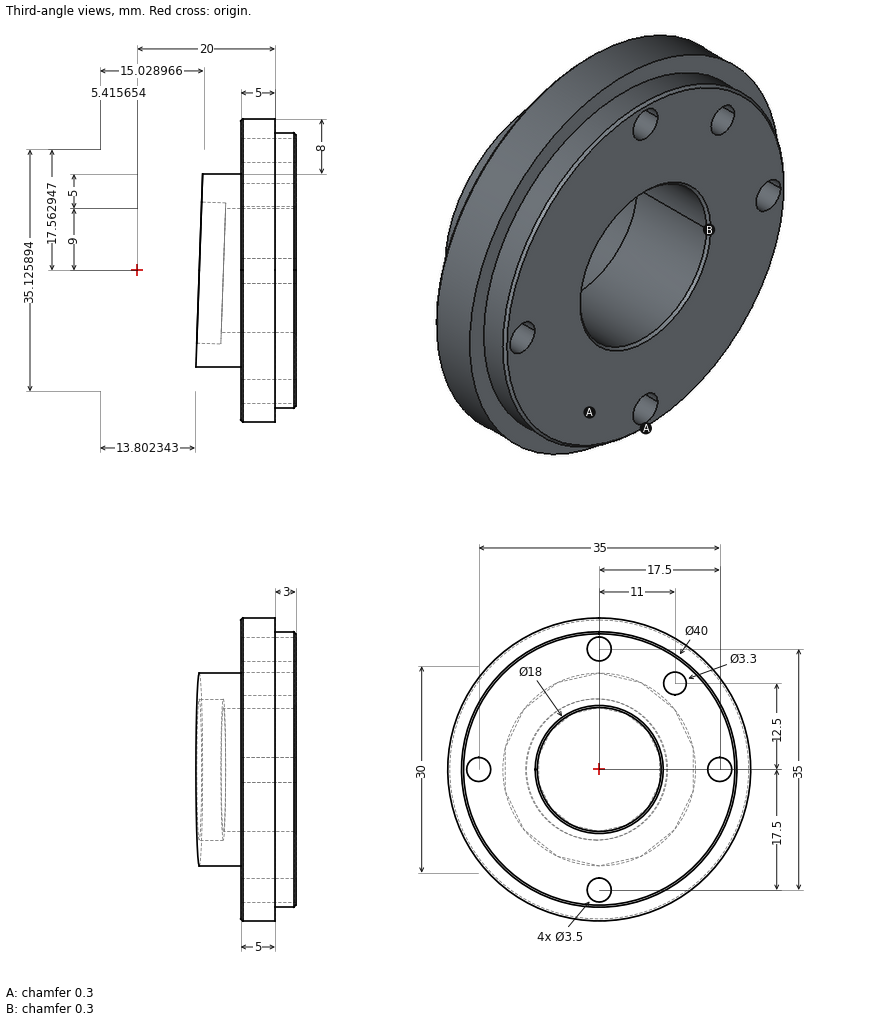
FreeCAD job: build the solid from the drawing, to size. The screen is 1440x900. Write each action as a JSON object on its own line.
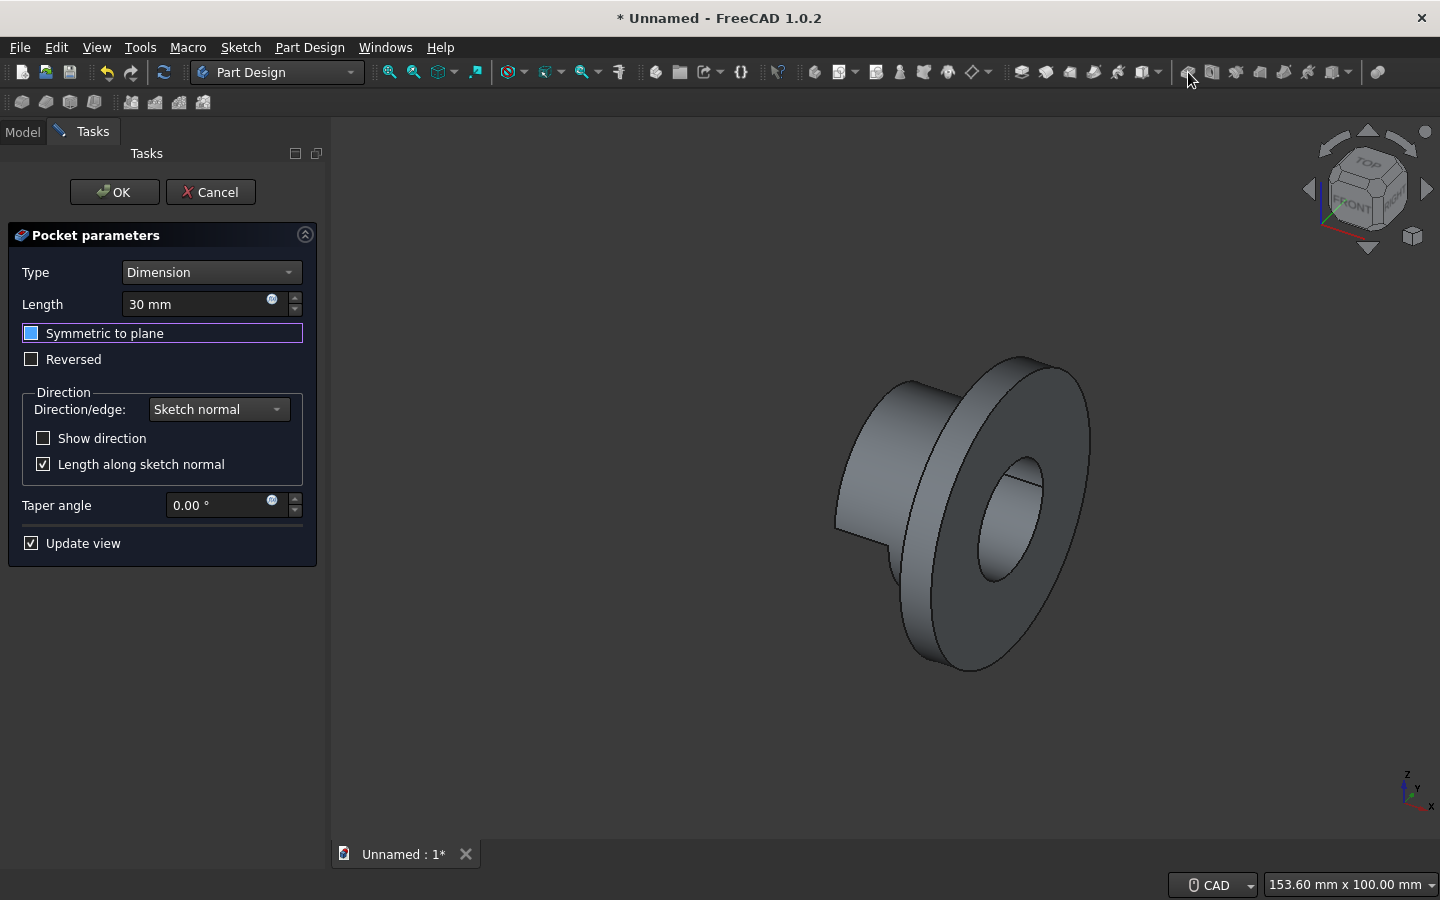
{"action": "left_click", "coordinate": [30, 333]}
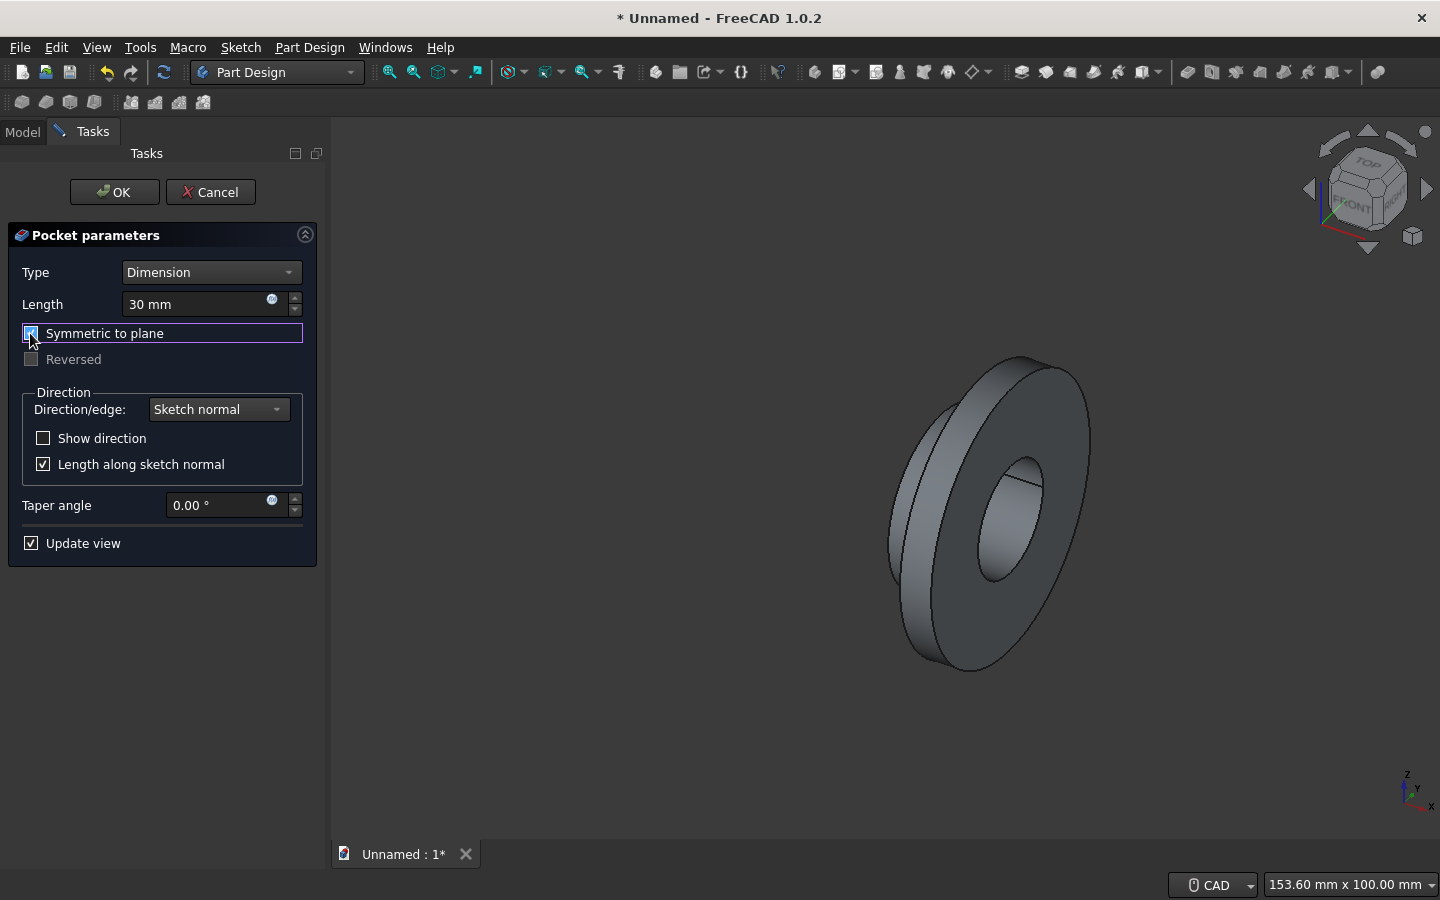
{"action": "left_click", "coordinate": [115, 192]}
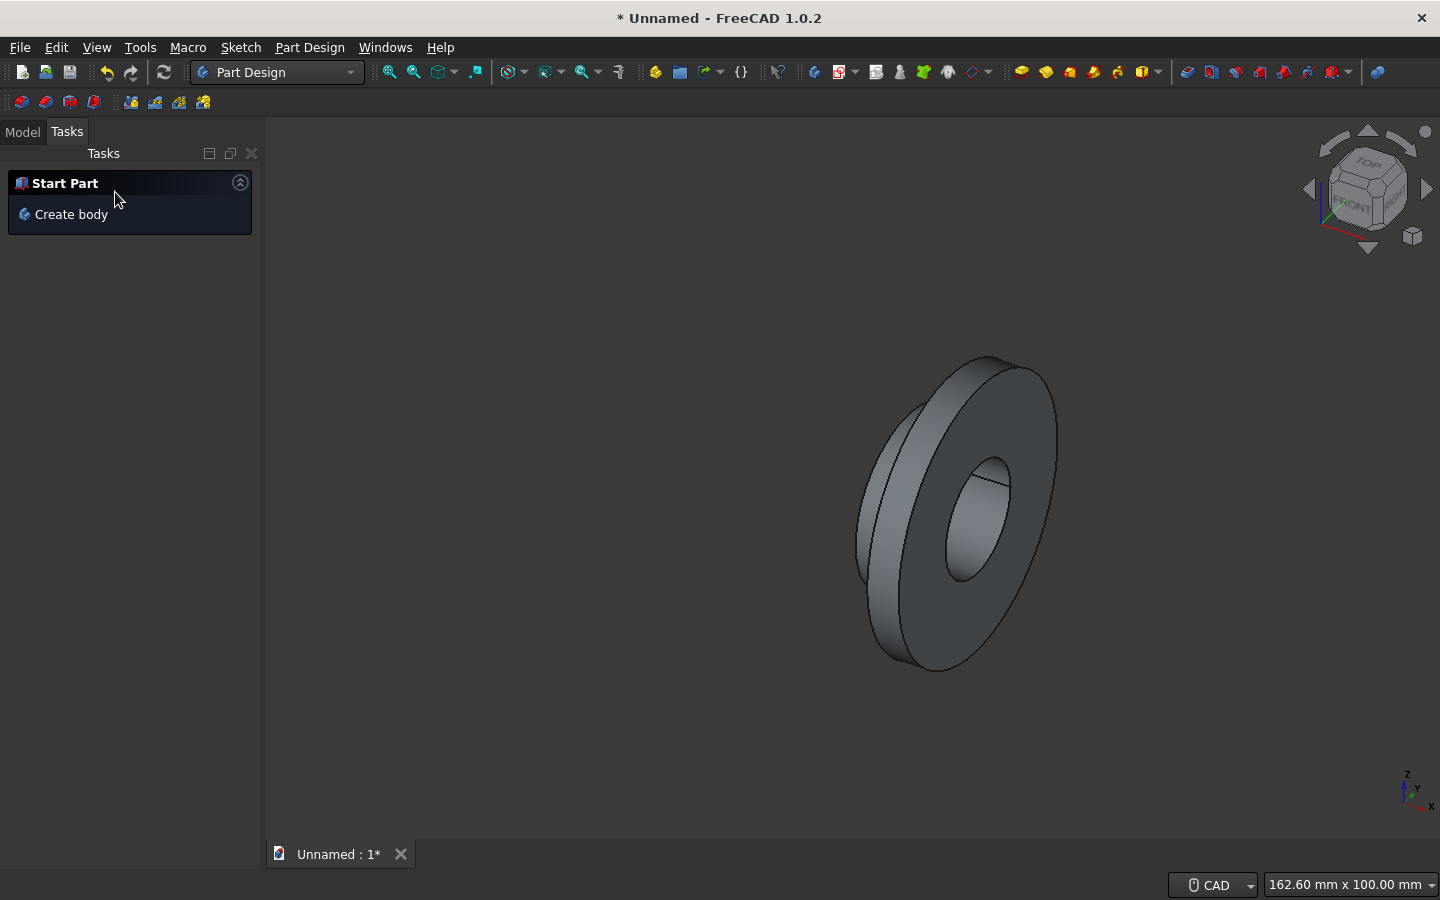
{"action": "key", "text": "6"}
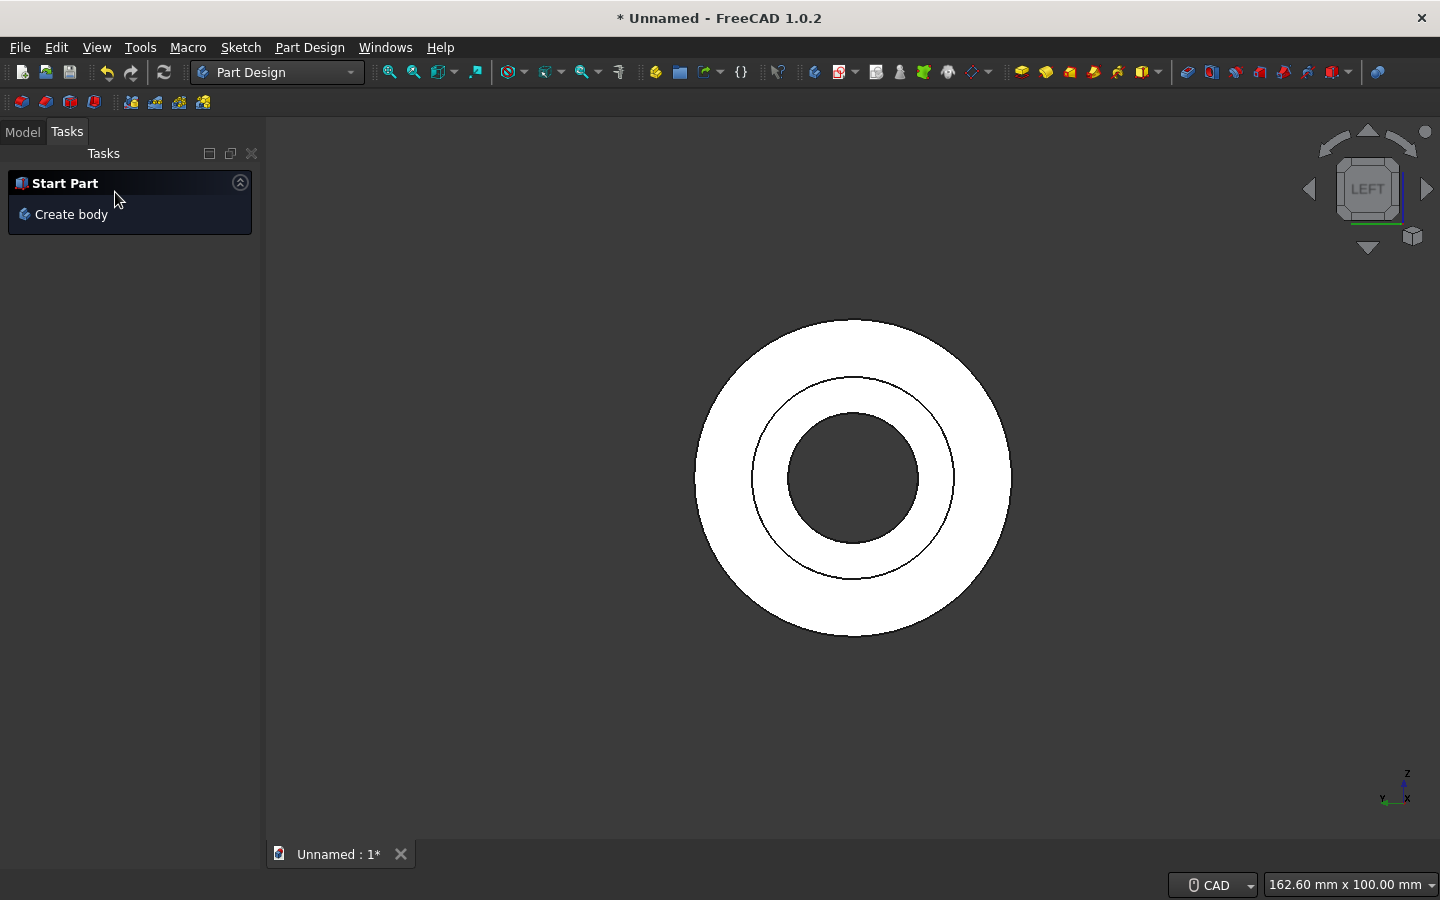
{"action": "key", "text": "v f"}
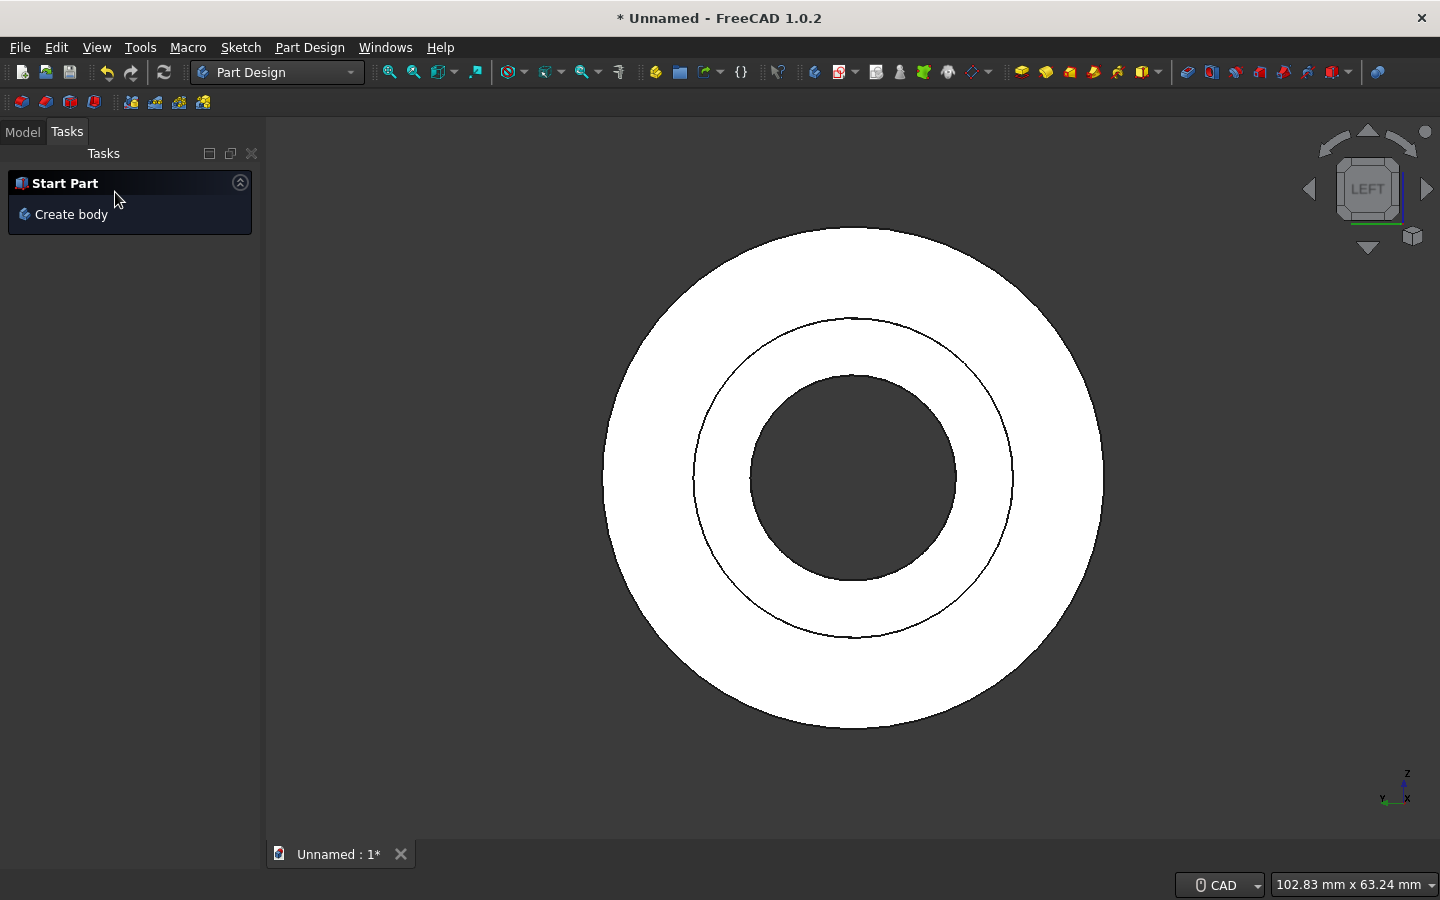
{"action": "left_click", "coordinate": [762, 386]}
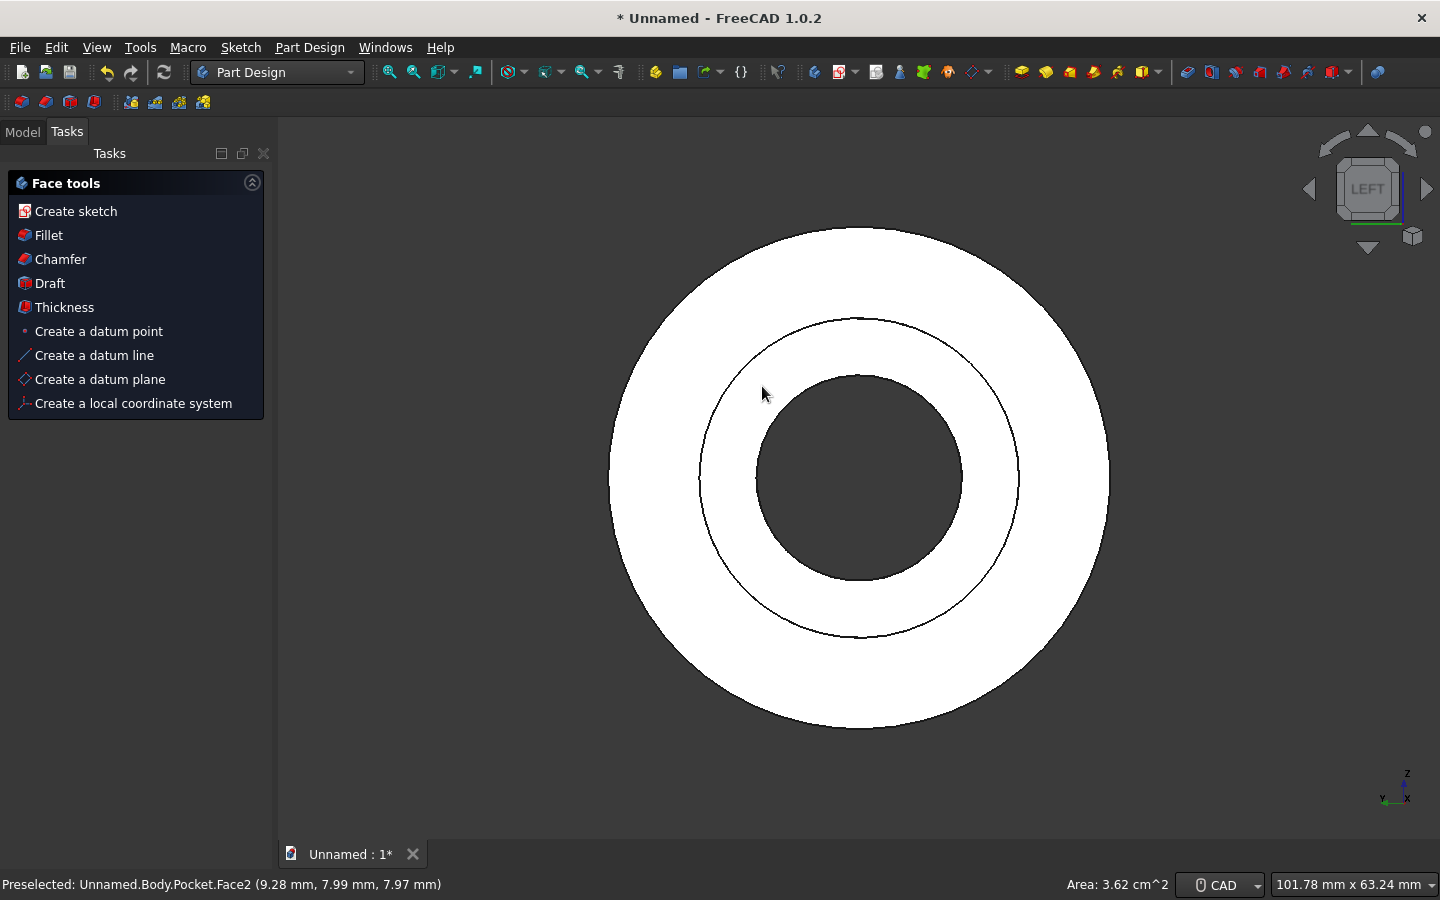
{"action": "left_click", "coordinate": [840, 72]}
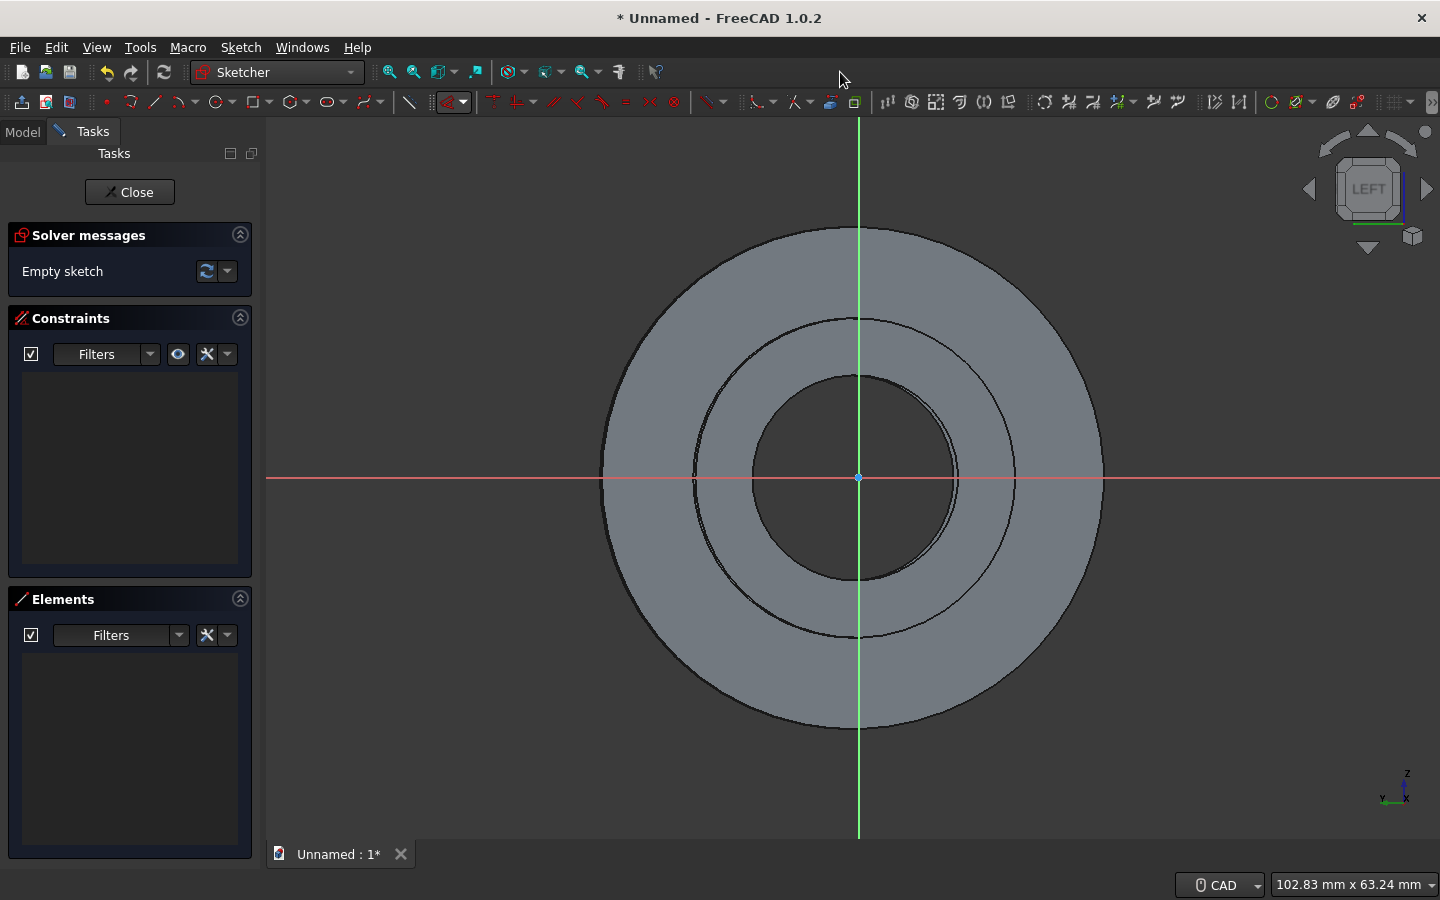
{"action": "key", "text": "q s"}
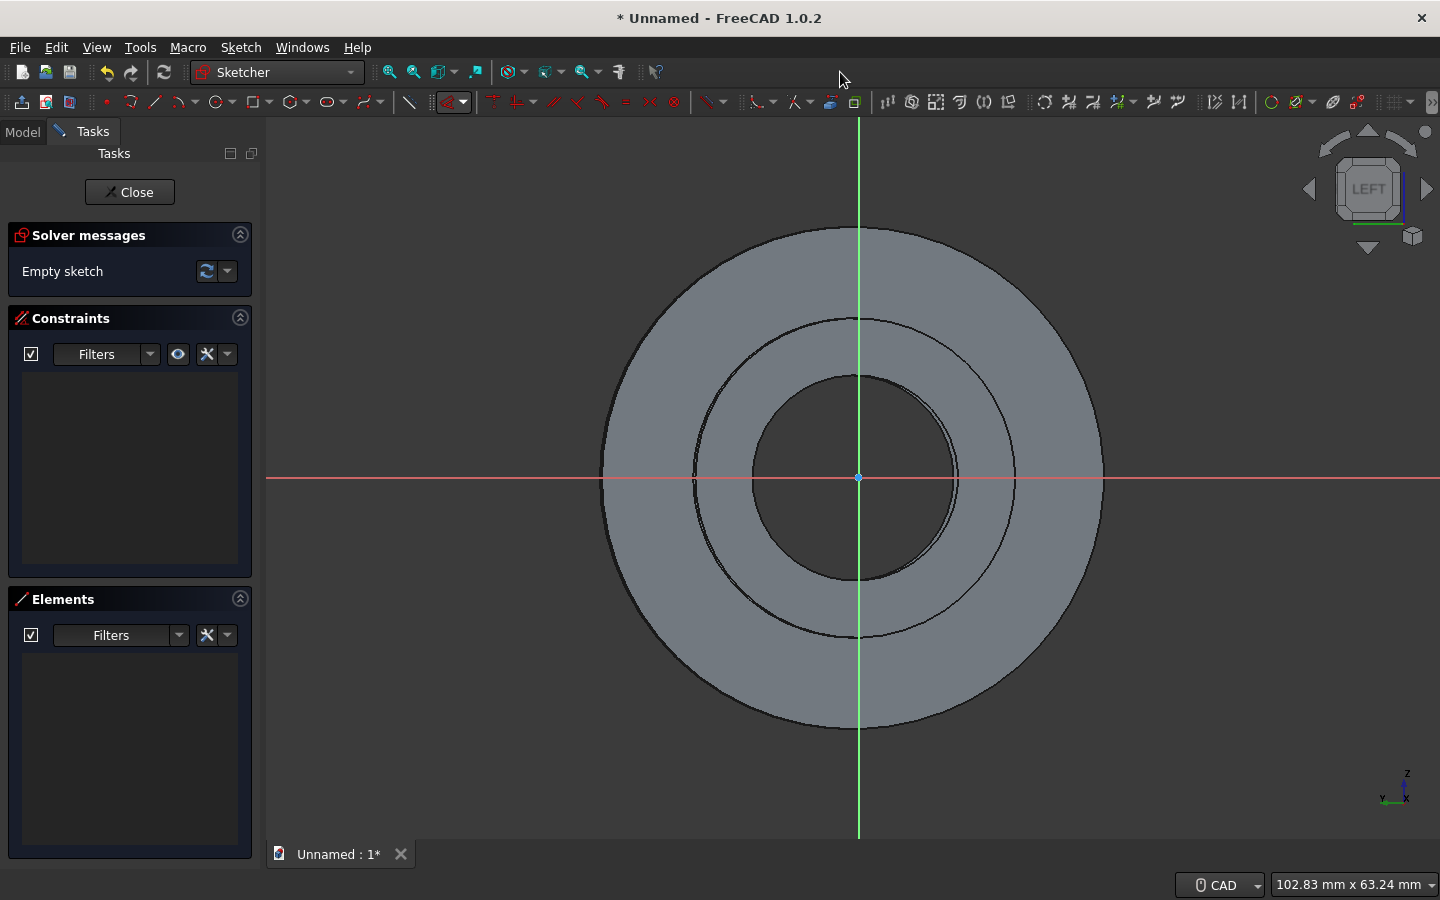
{"action": "scroll", "coordinate": [949, 478], "scroll_direction": "up", "scroll_amount": 3}